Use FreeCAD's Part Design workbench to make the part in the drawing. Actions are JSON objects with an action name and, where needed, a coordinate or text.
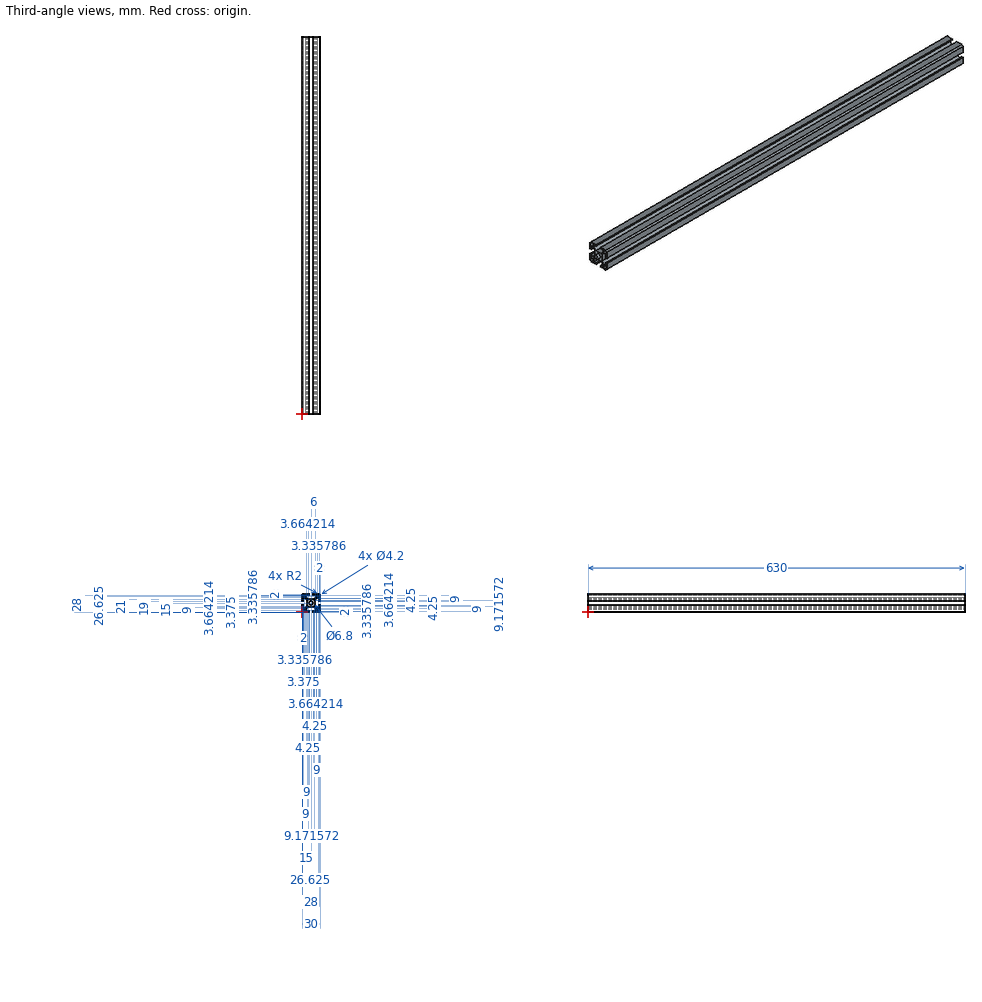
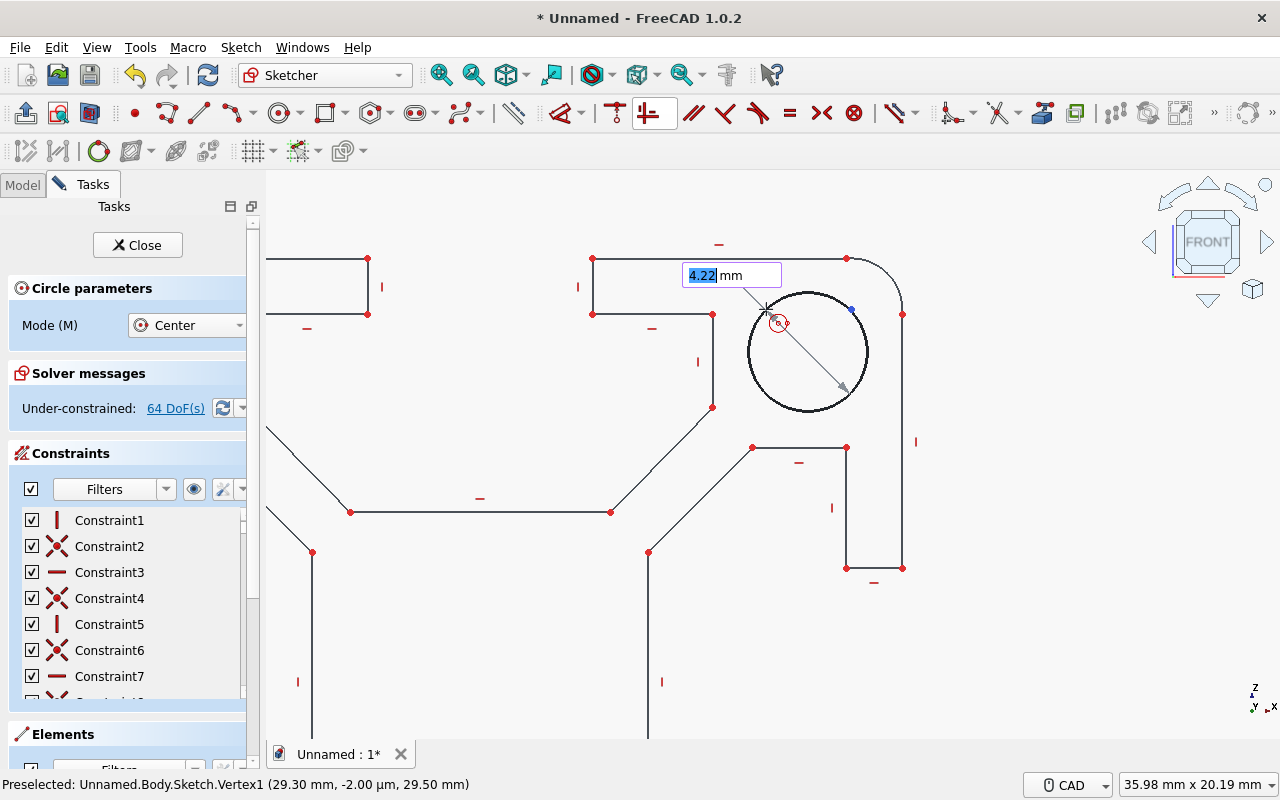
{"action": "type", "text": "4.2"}
{"action": "key", "text": "Return"}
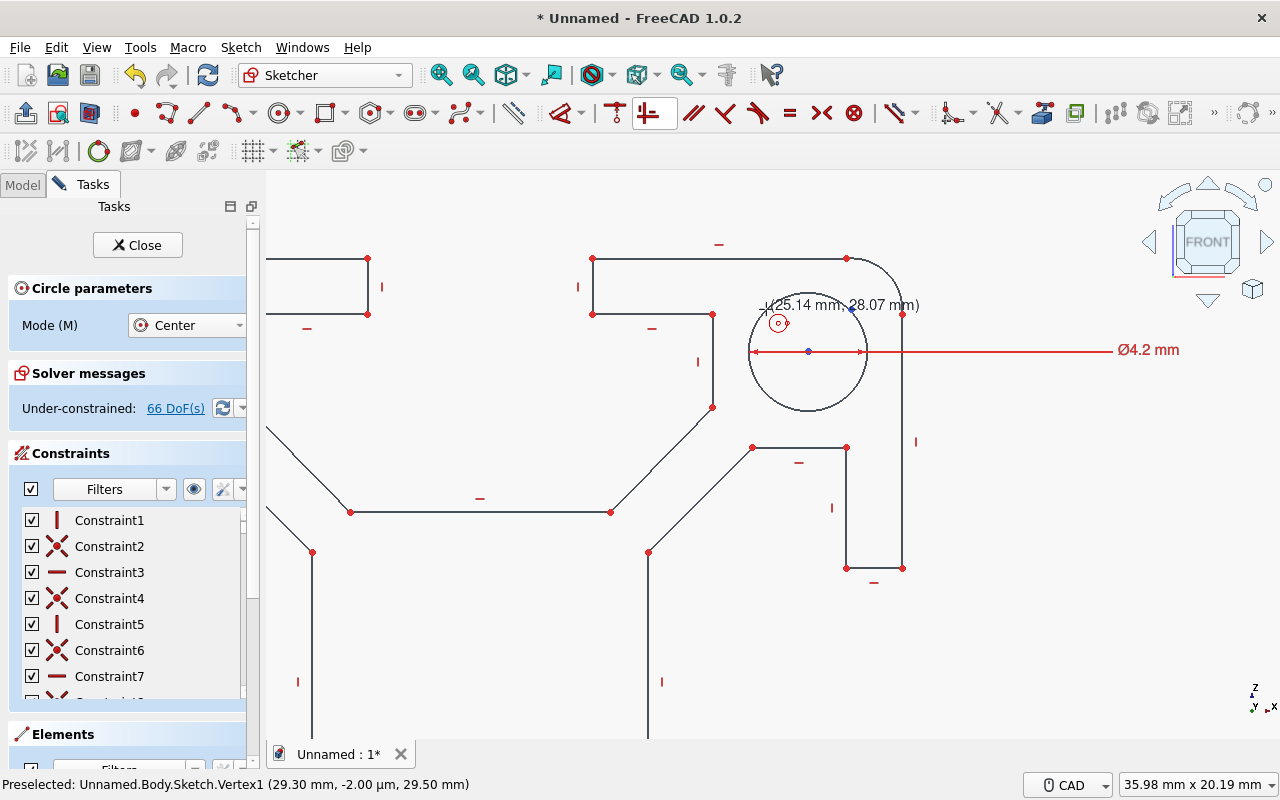
{"action": "scroll", "coordinate": [887, 272], "scroll_direction": "down", "scroll_amount": 4}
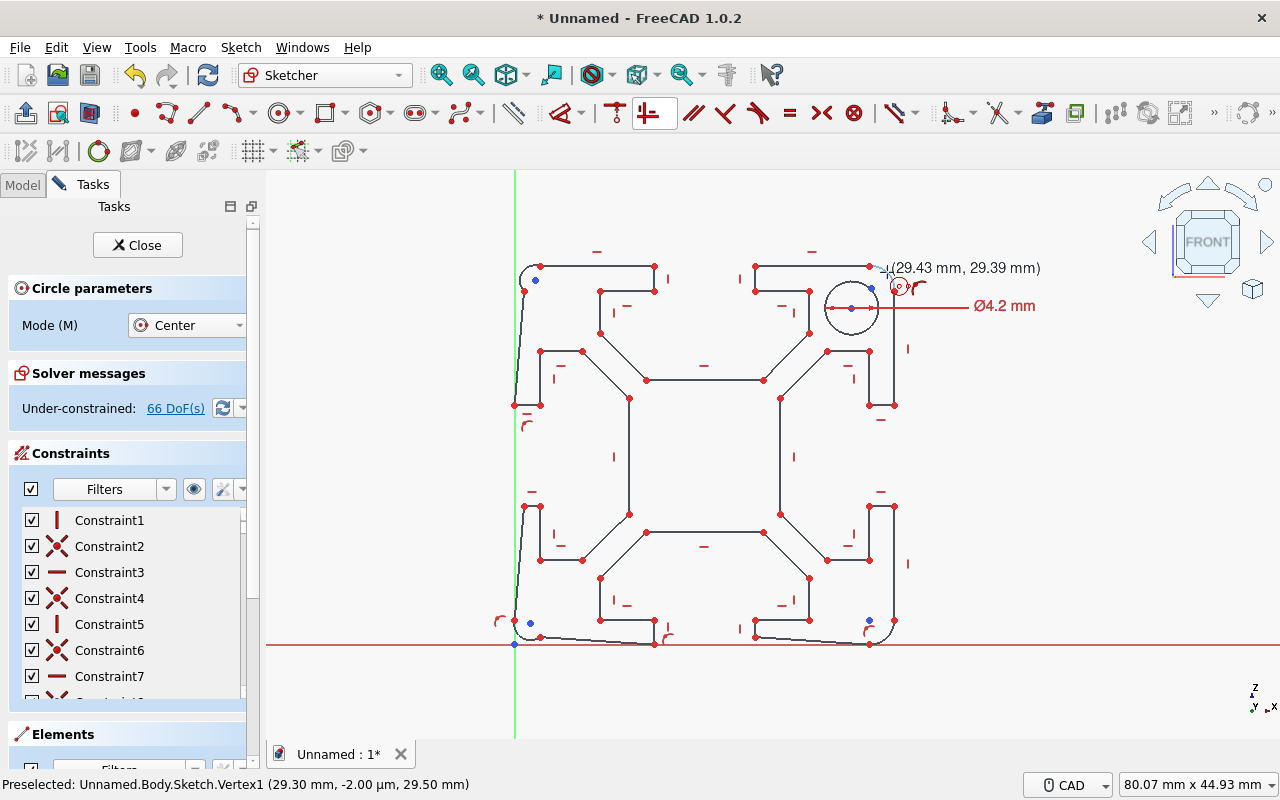
{"action": "left_click", "coordinate": [557, 308]}
{"action": "mouse_move", "coordinate": [576, 289]}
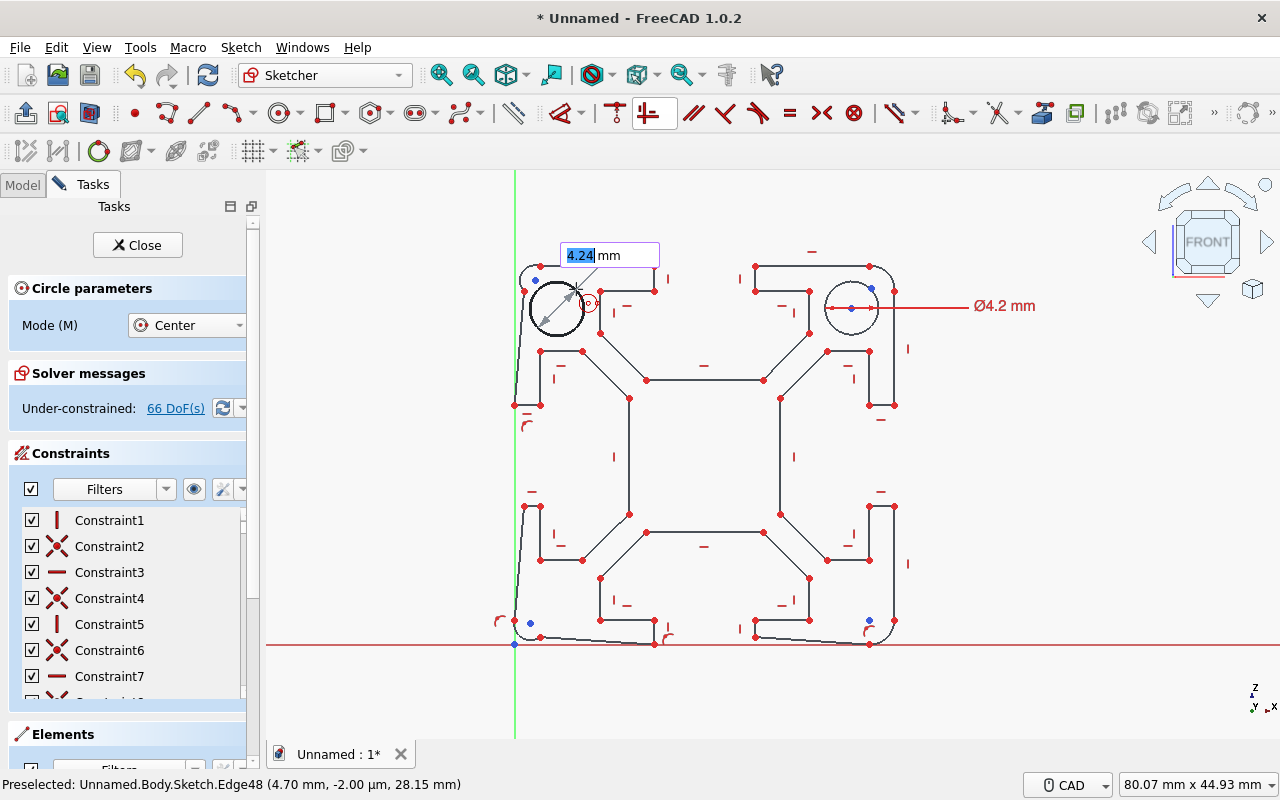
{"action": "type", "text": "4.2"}
{"action": "key", "text": "Return"}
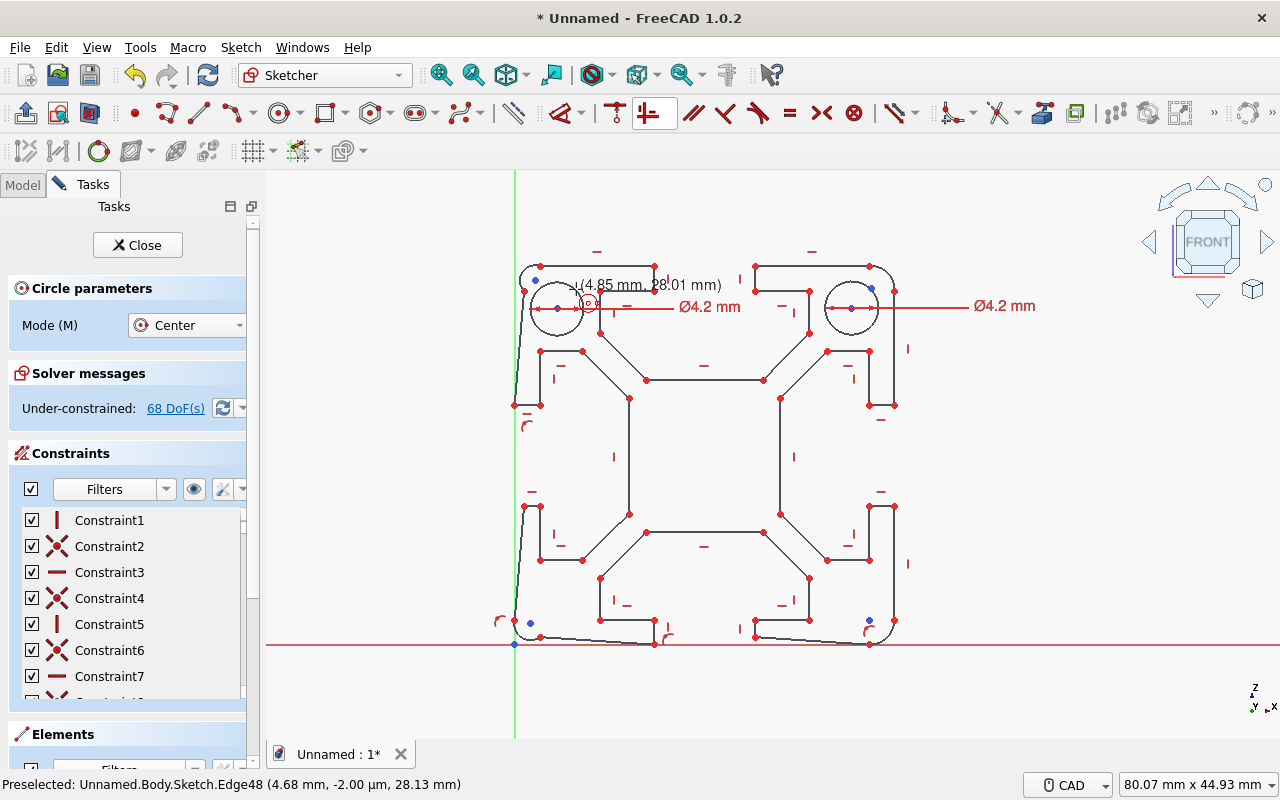
{"action": "left_click", "coordinate": [852, 602]}
{"action": "mouse_move", "coordinate": [871, 583]}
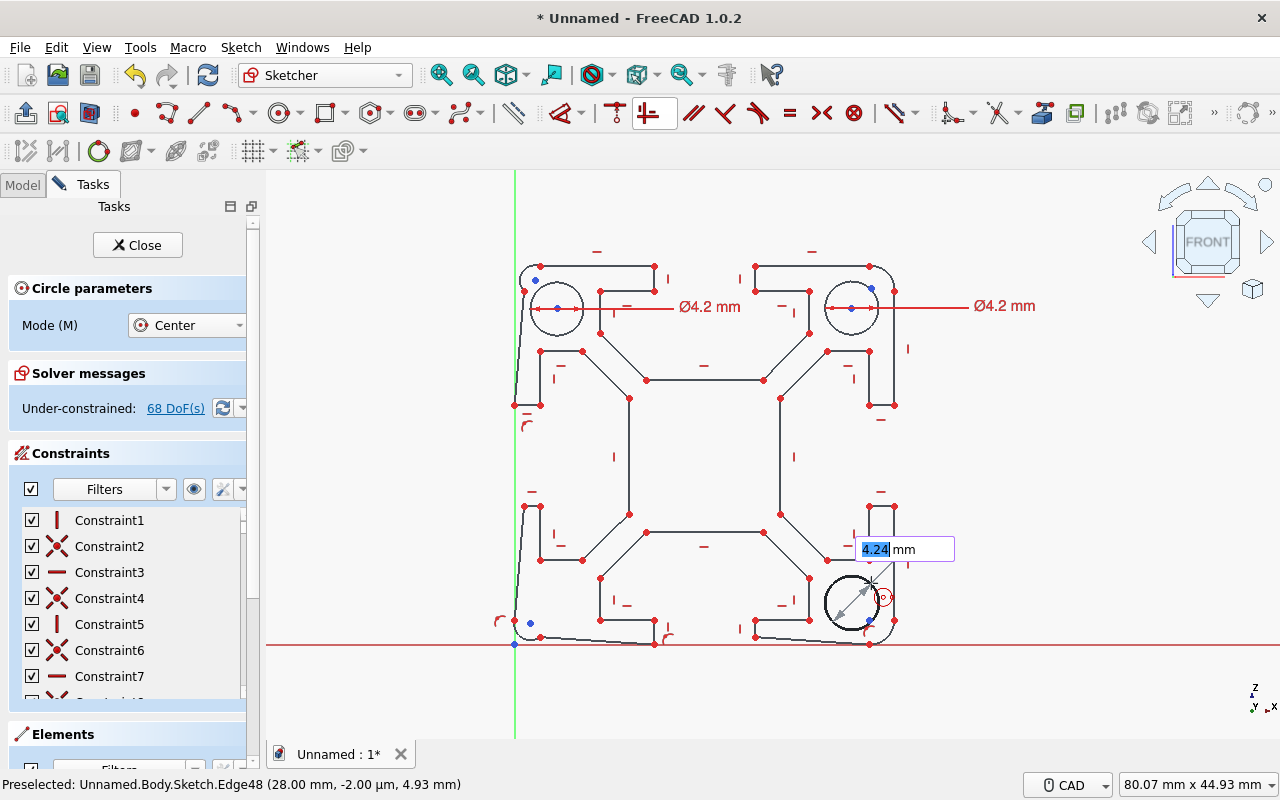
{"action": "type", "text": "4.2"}
{"action": "key", "text": "Return"}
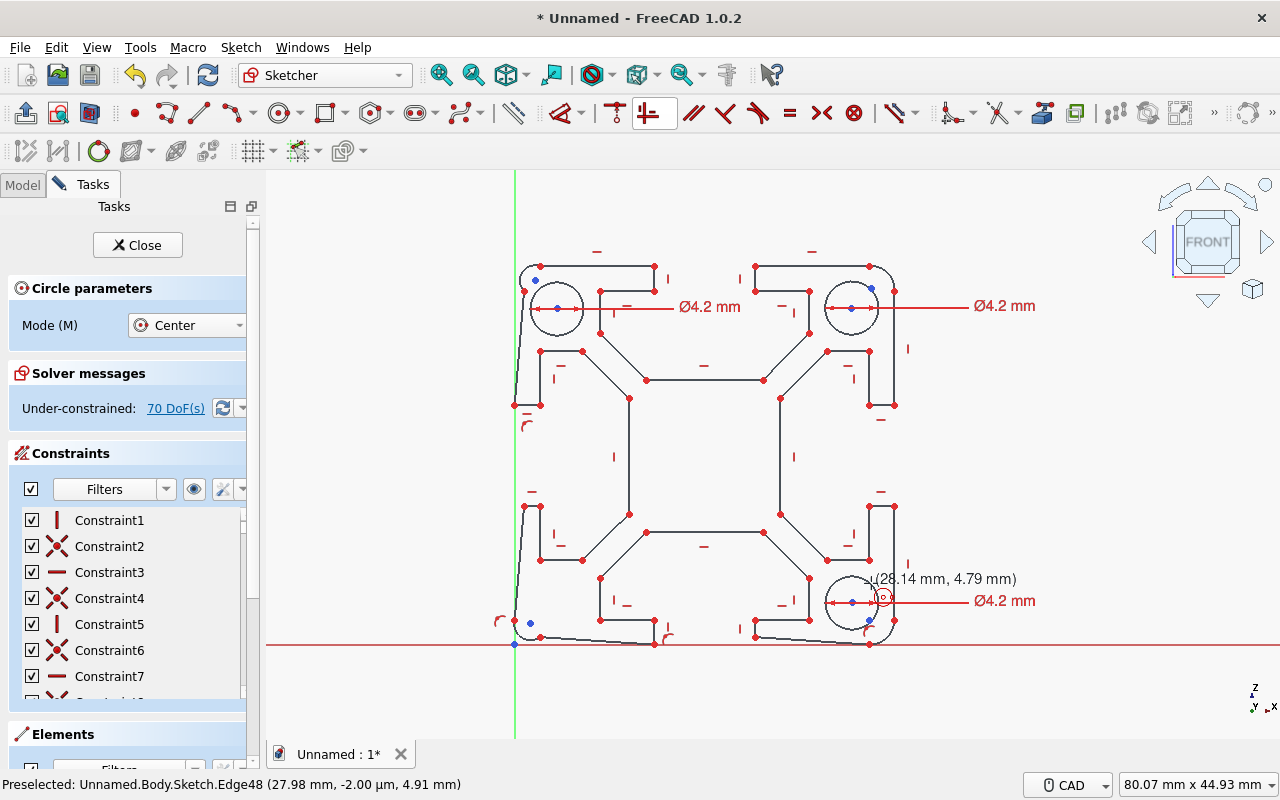
{"action": "left_click", "coordinate": [705, 455]}
{"action": "mouse_move", "coordinate": [735, 424]}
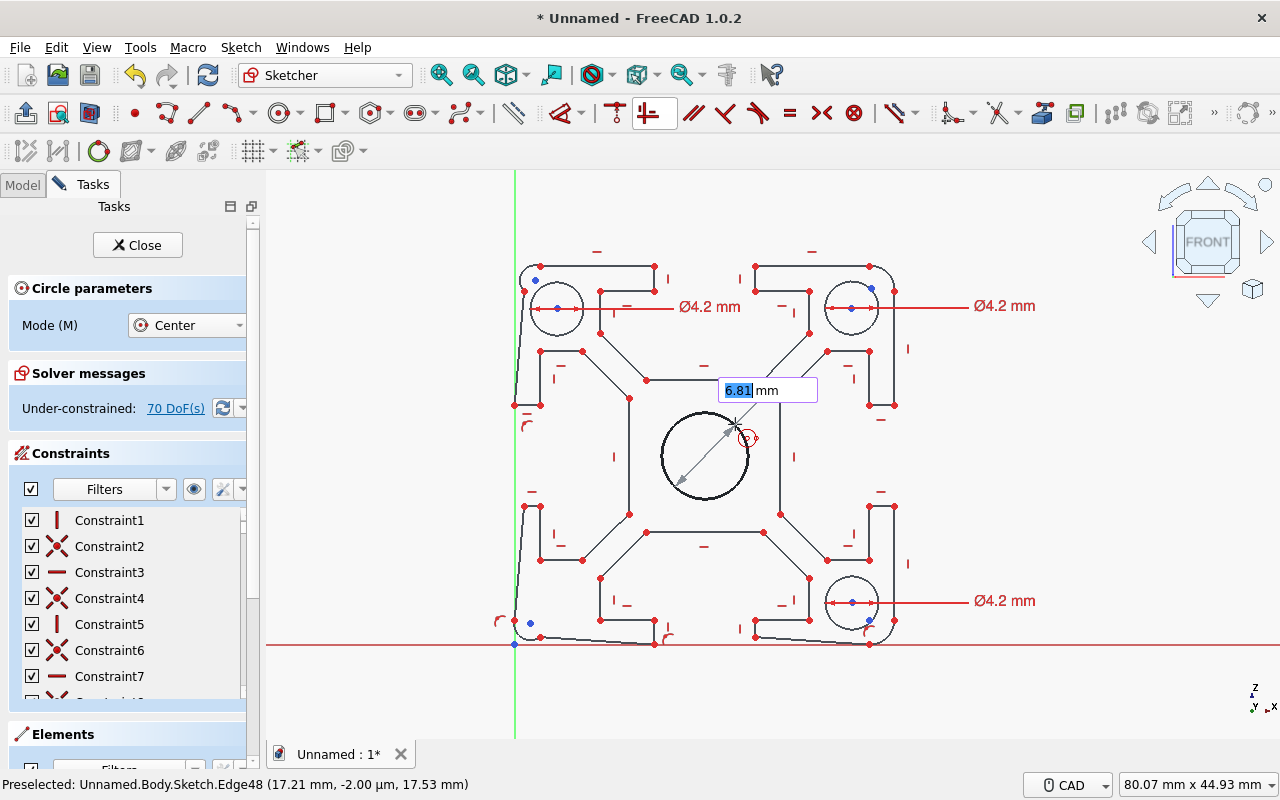
{"action": "type", "text": "6.8"}
{"action": "key", "text": "Return"}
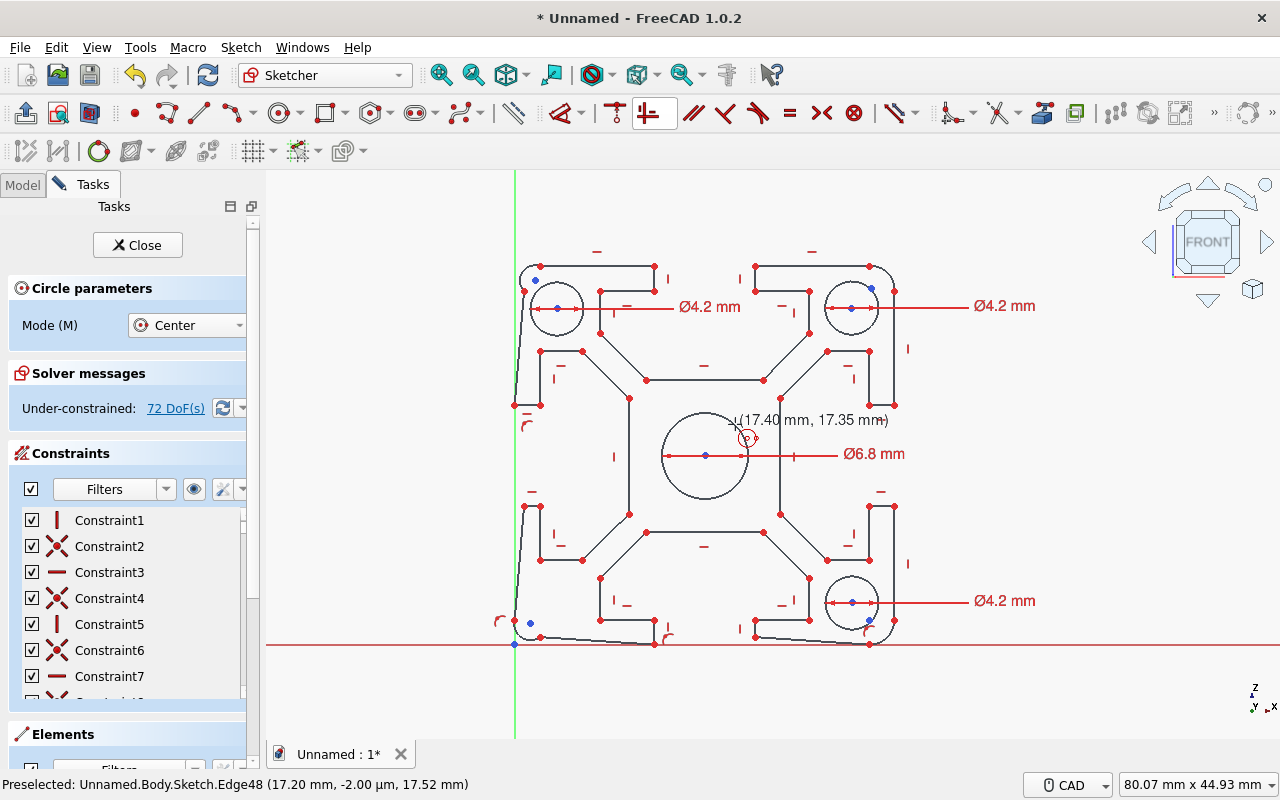
{"action": "left_click", "coordinate": [557, 602]}
{"action": "mouse_move", "coordinate": [576, 583]}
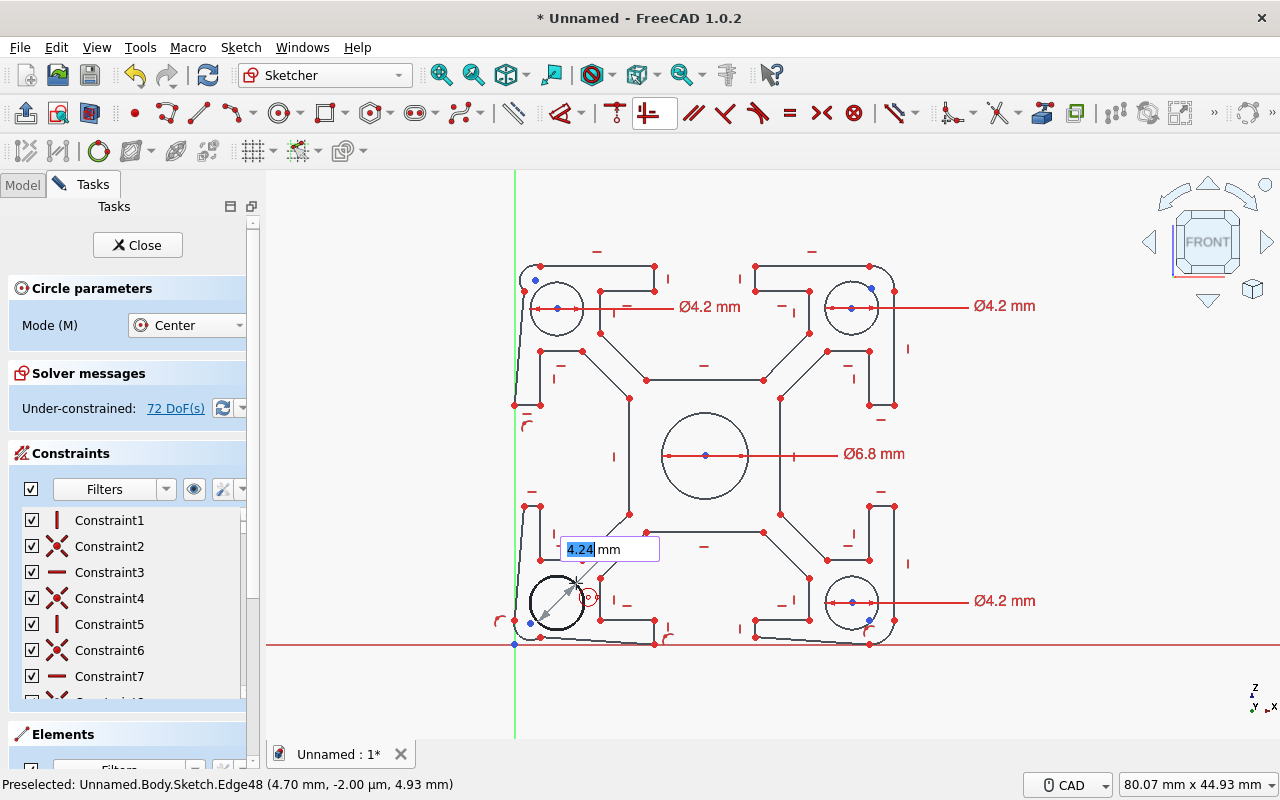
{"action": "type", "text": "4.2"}
{"action": "key", "text": "Return"}
{"action": "key", "text": "Escape"}